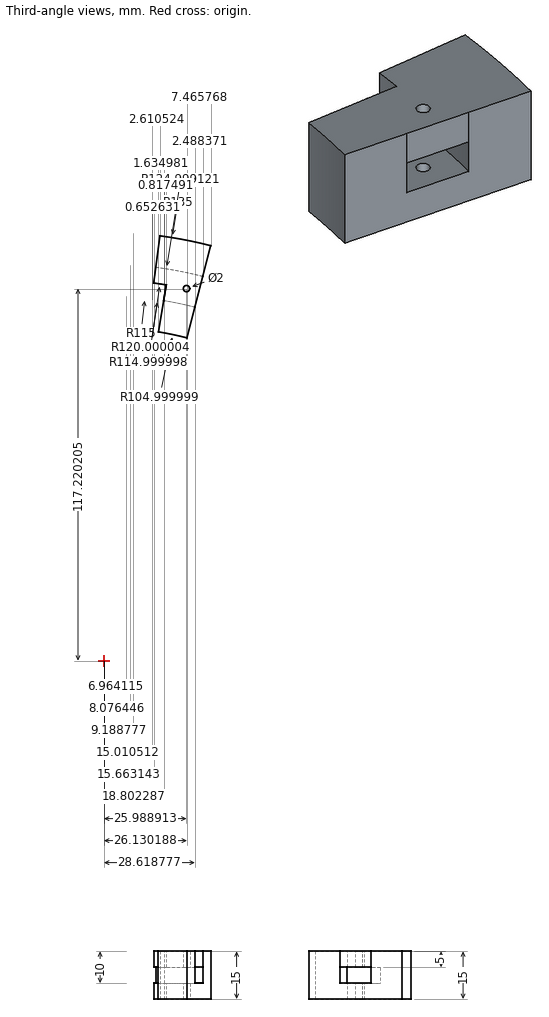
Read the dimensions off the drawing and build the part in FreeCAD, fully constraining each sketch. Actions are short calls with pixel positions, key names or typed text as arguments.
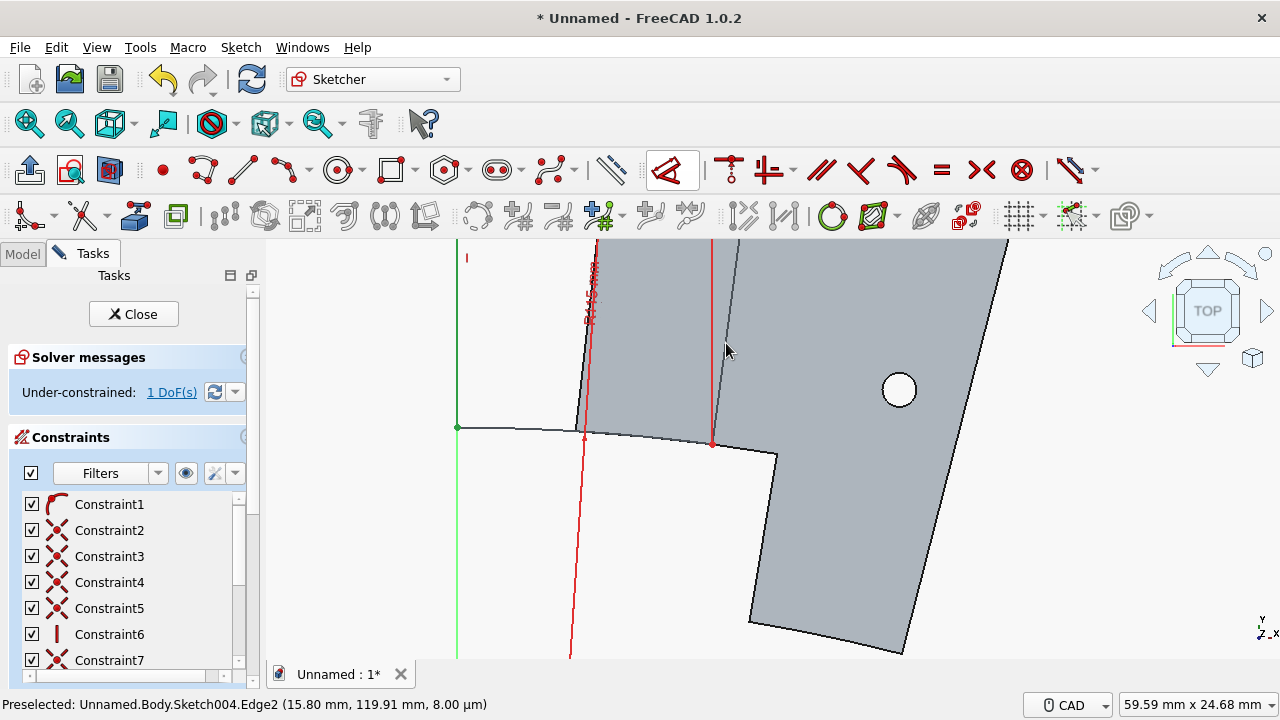
click(712, 444)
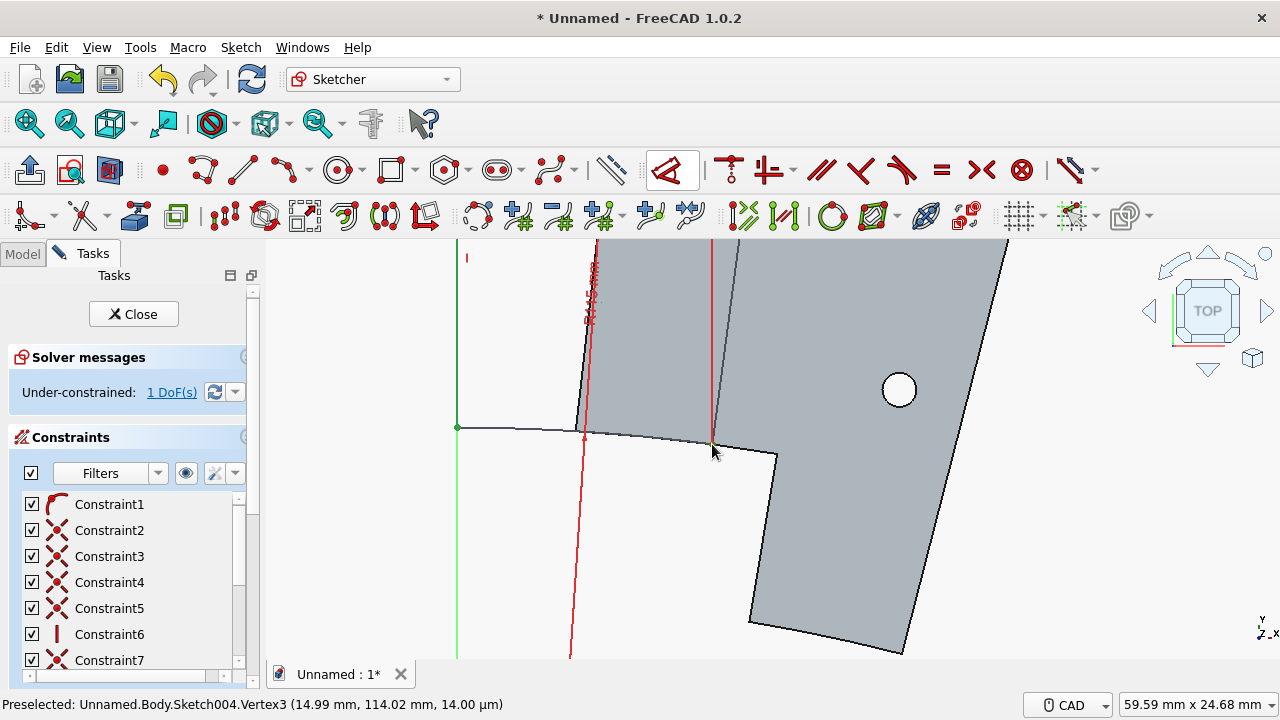
key(l)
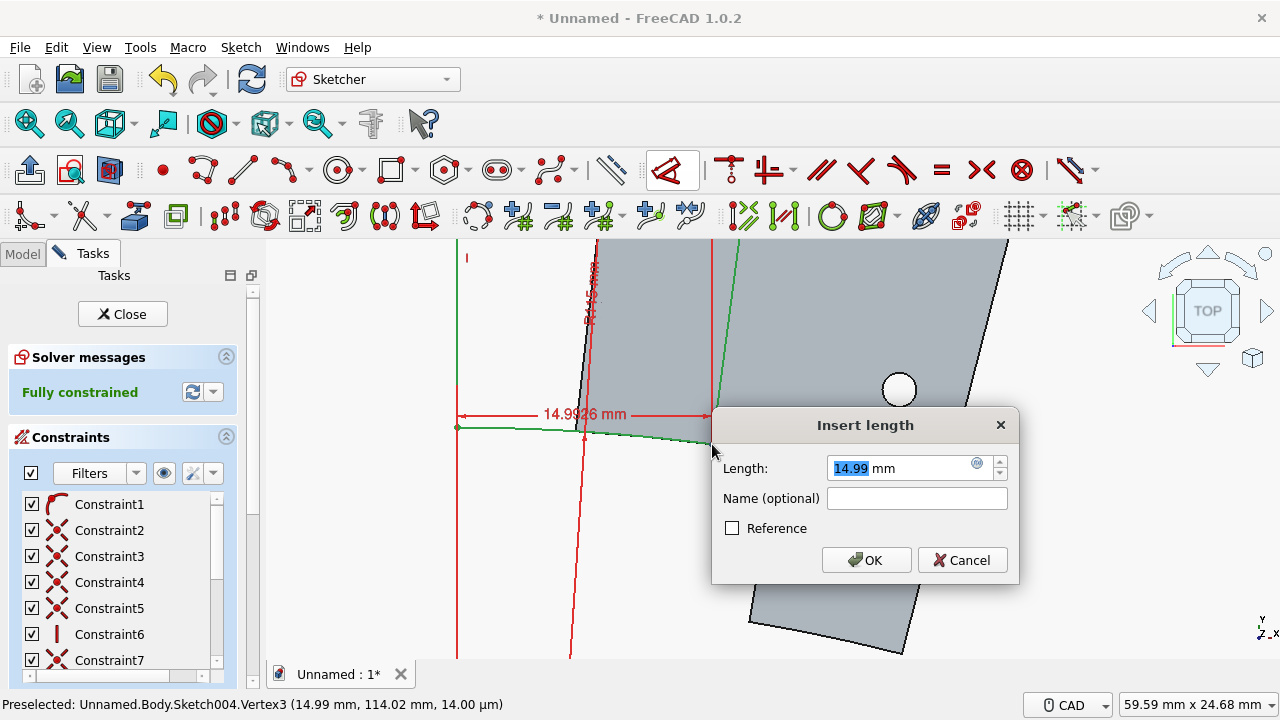
text(15.010512)
key(Return)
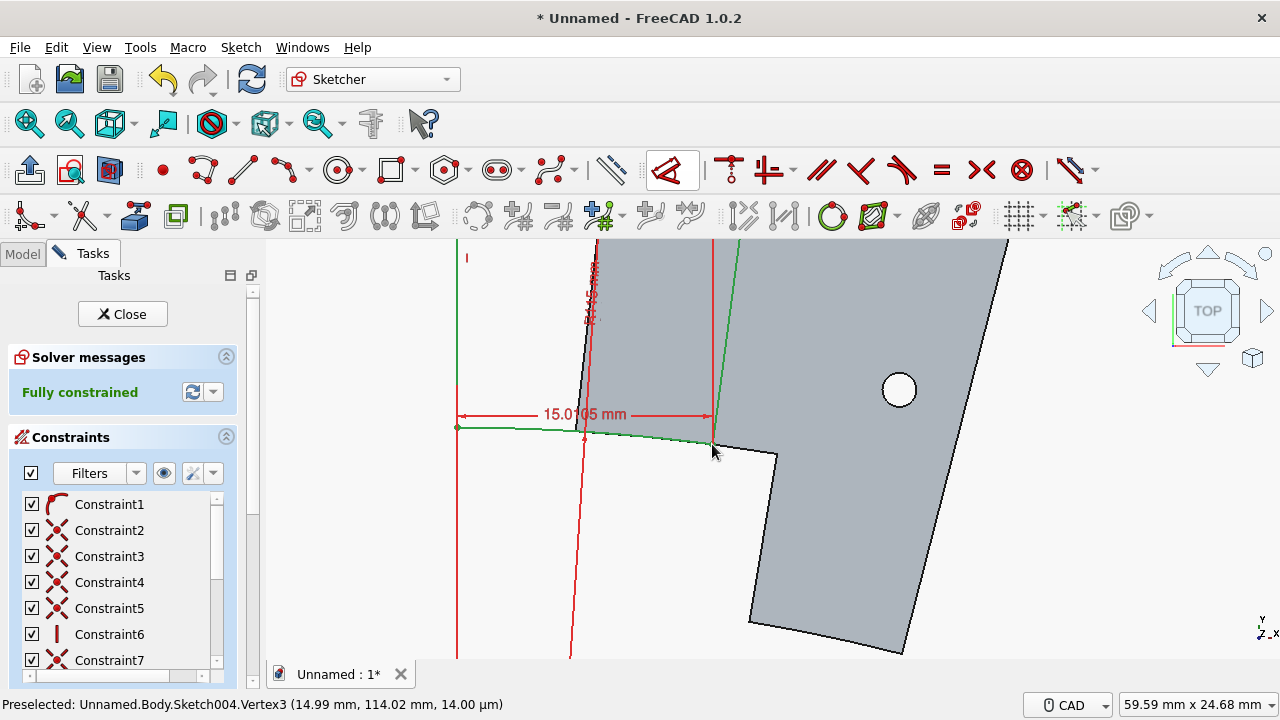
click(123, 314)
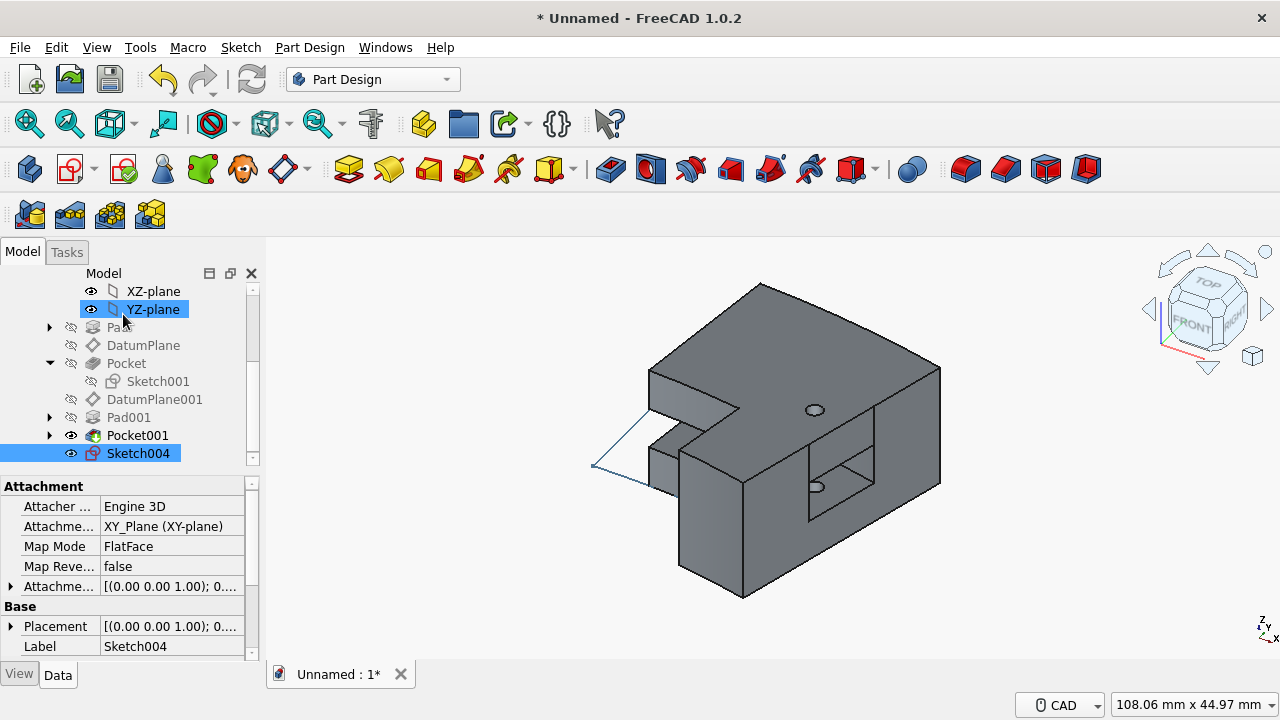
click(612, 170)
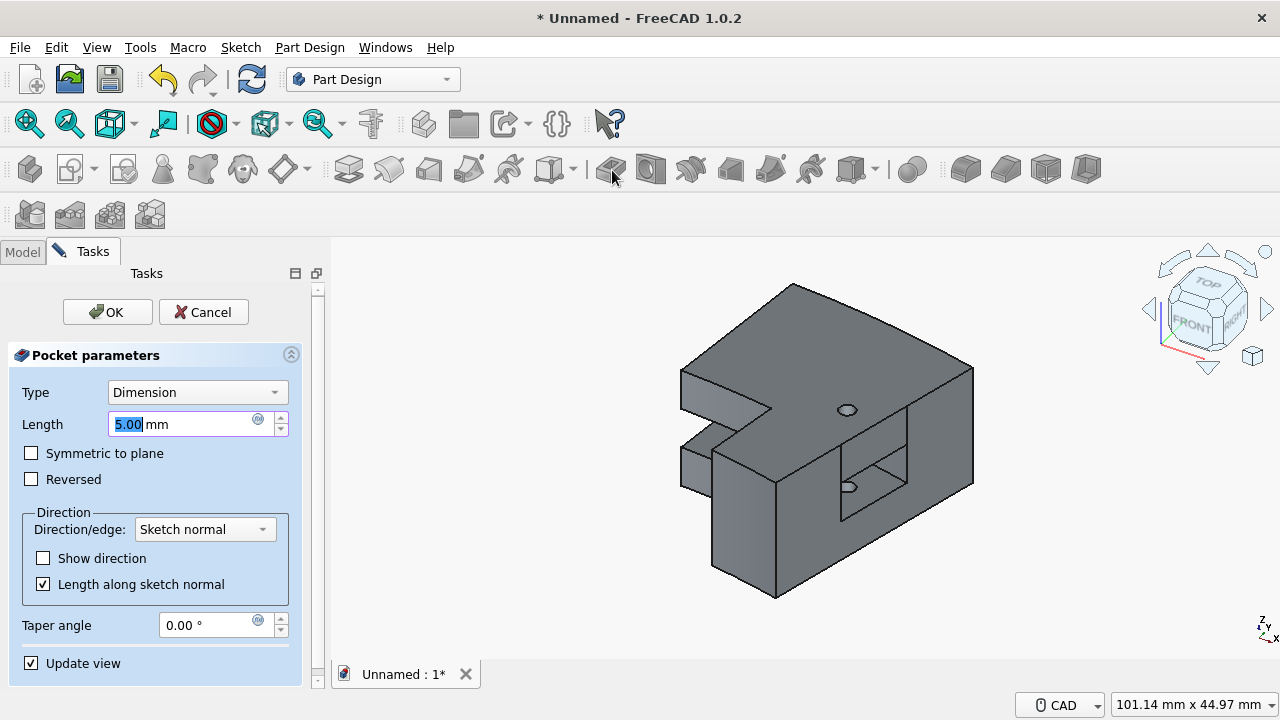
text(15)
key(Tab)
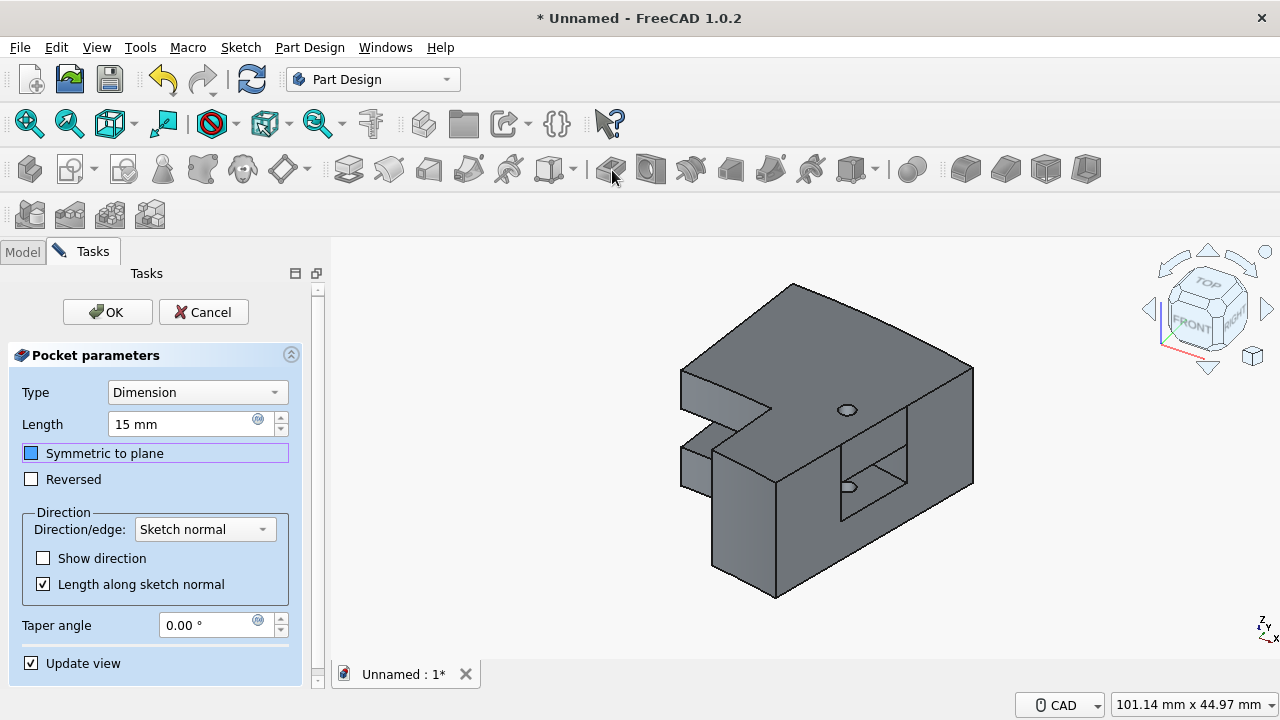
click(30, 479)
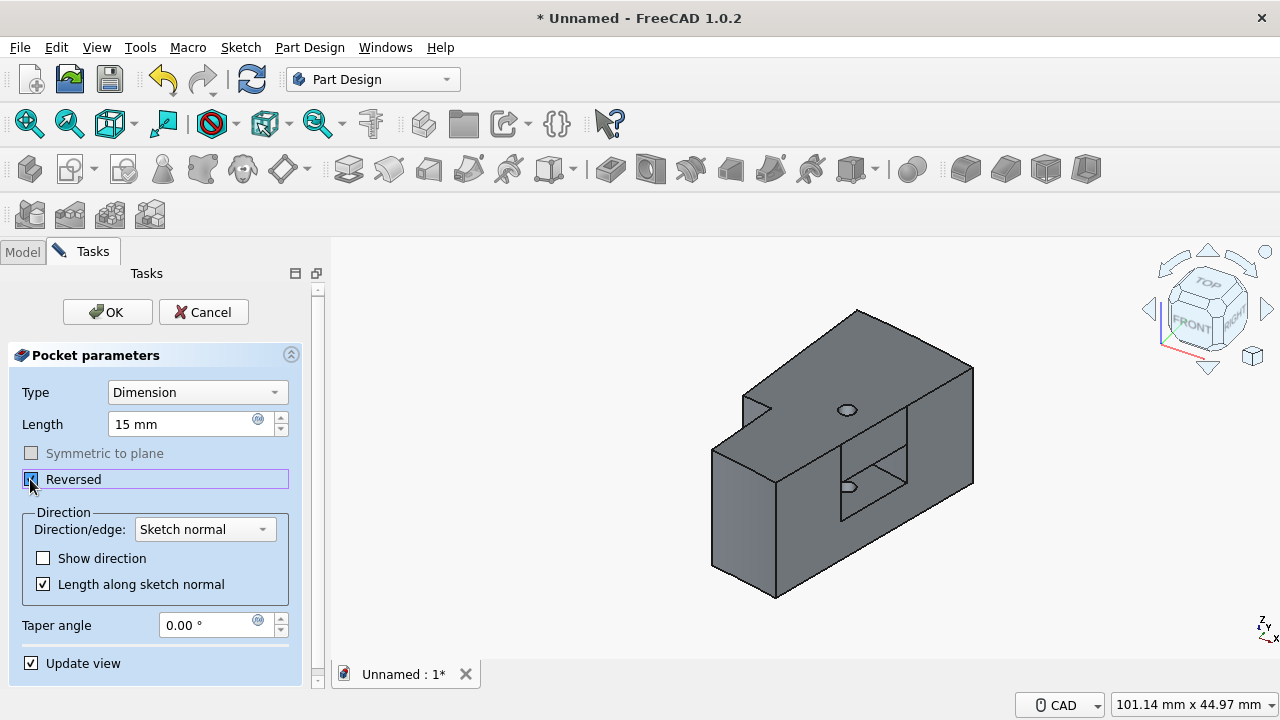
click(108, 312)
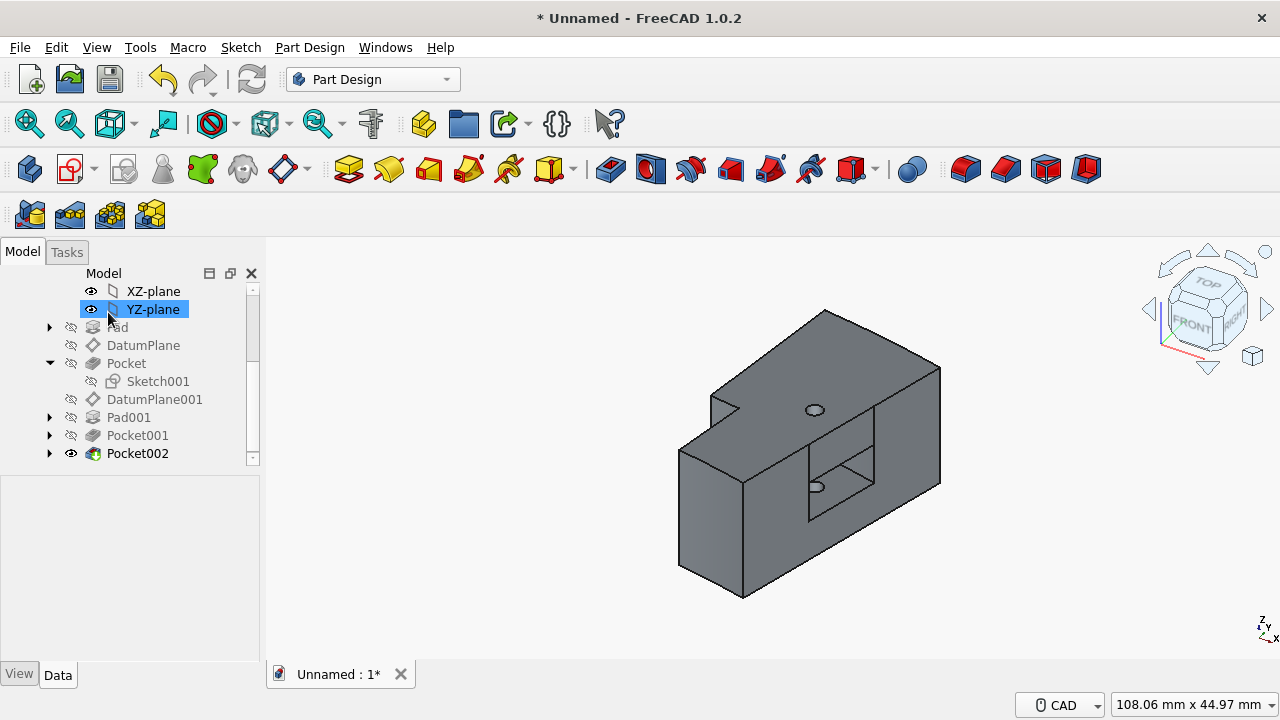
click(70, 170)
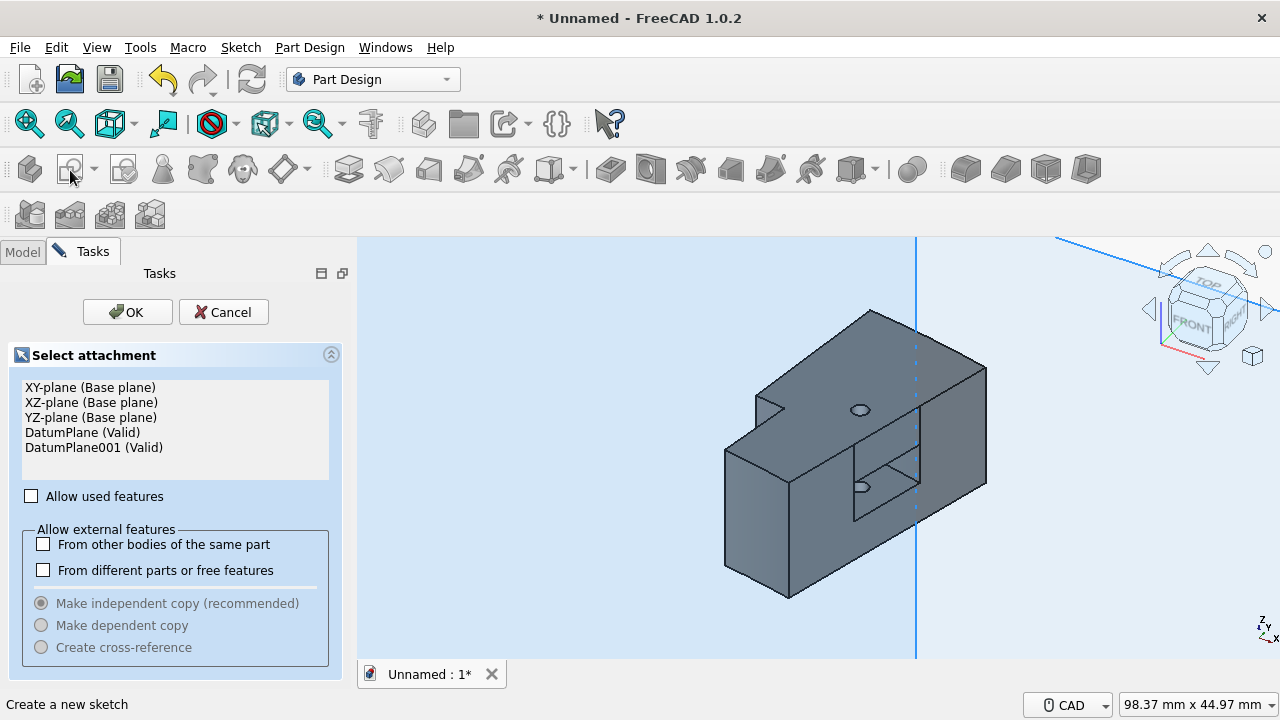
click(82, 388)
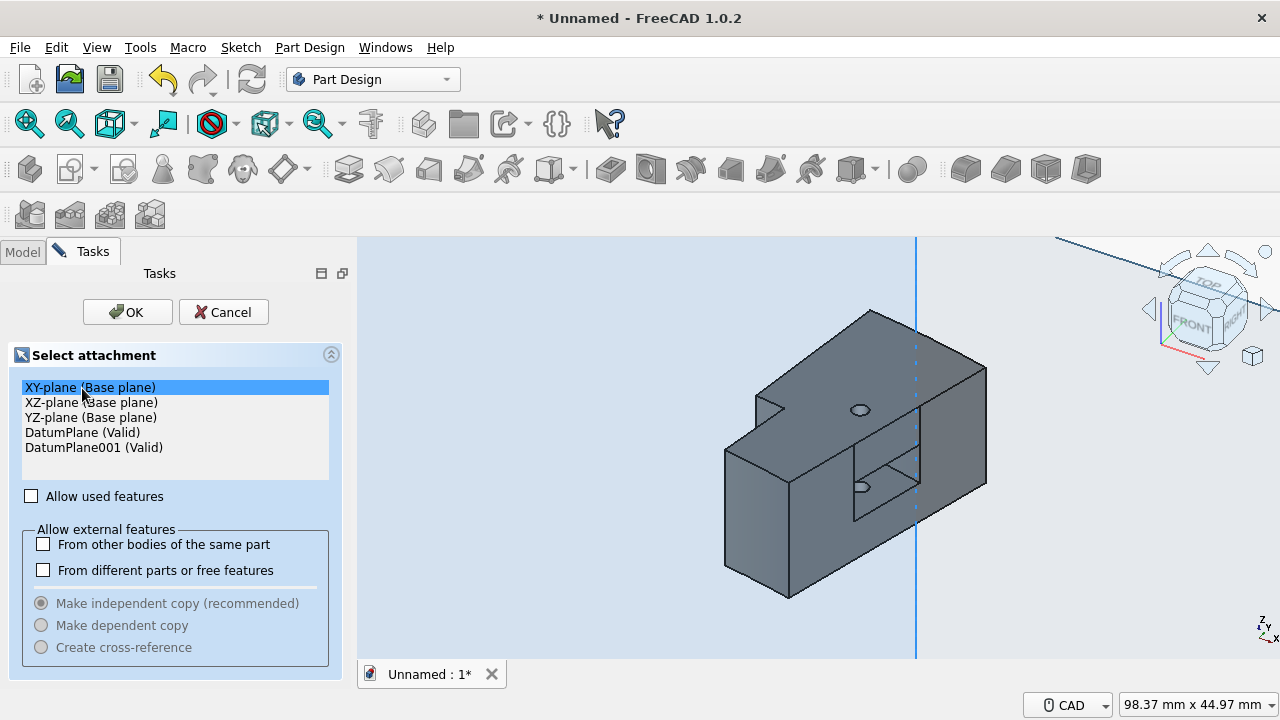
click(128, 312)